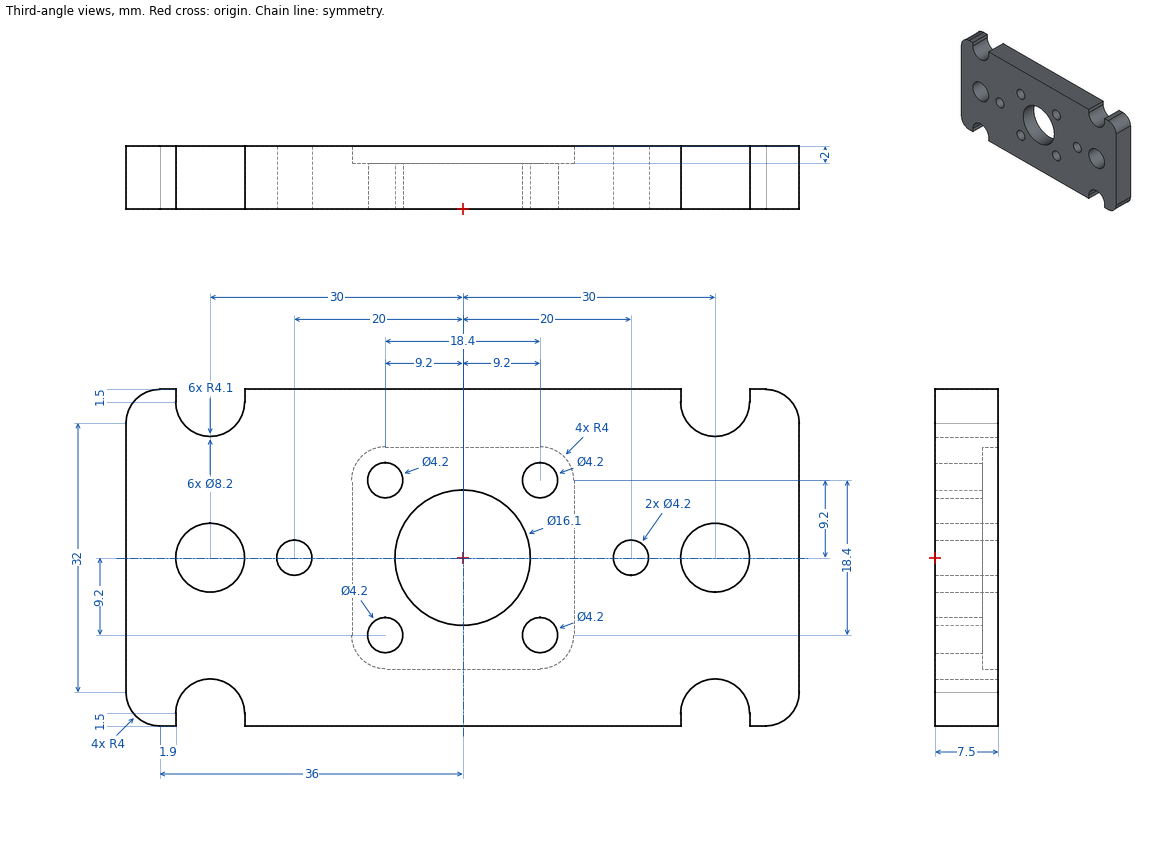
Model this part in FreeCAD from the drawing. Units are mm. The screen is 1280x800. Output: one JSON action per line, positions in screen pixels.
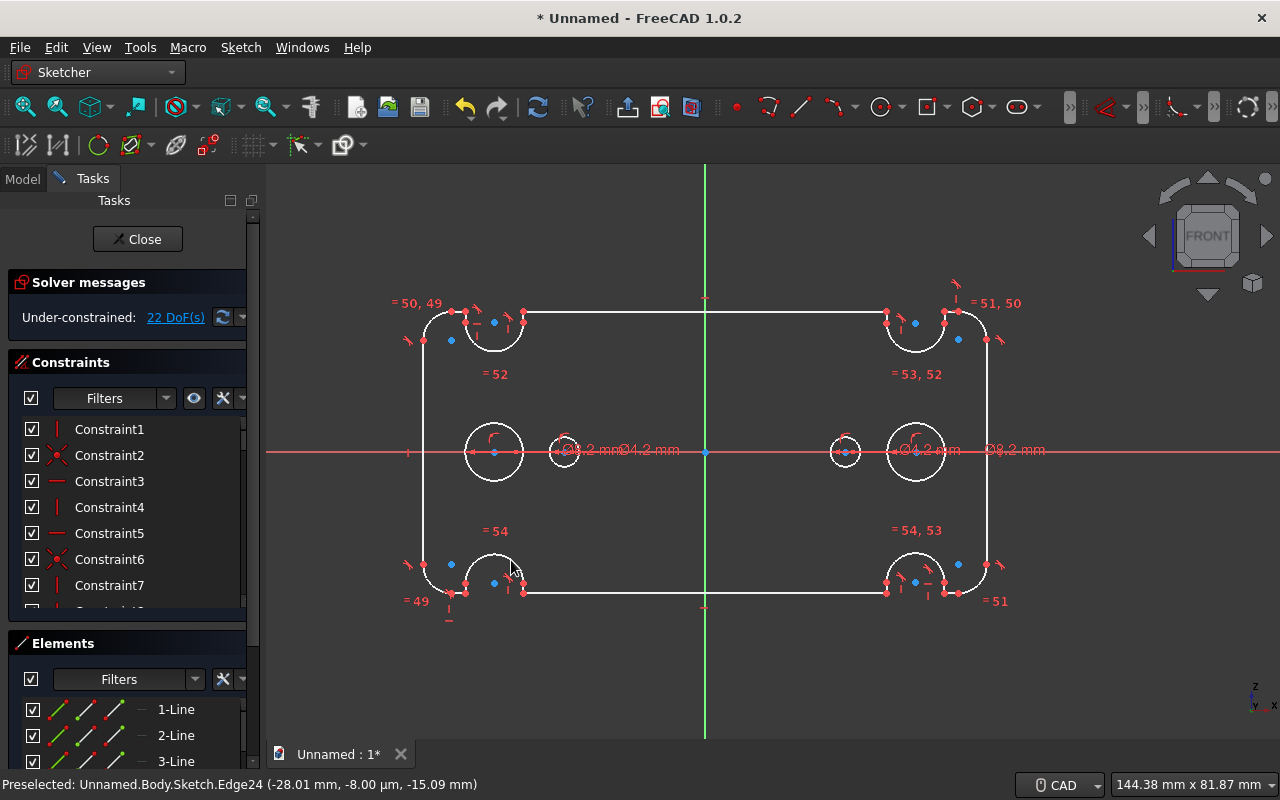
{"action": "left_click", "coordinate": [494, 323]}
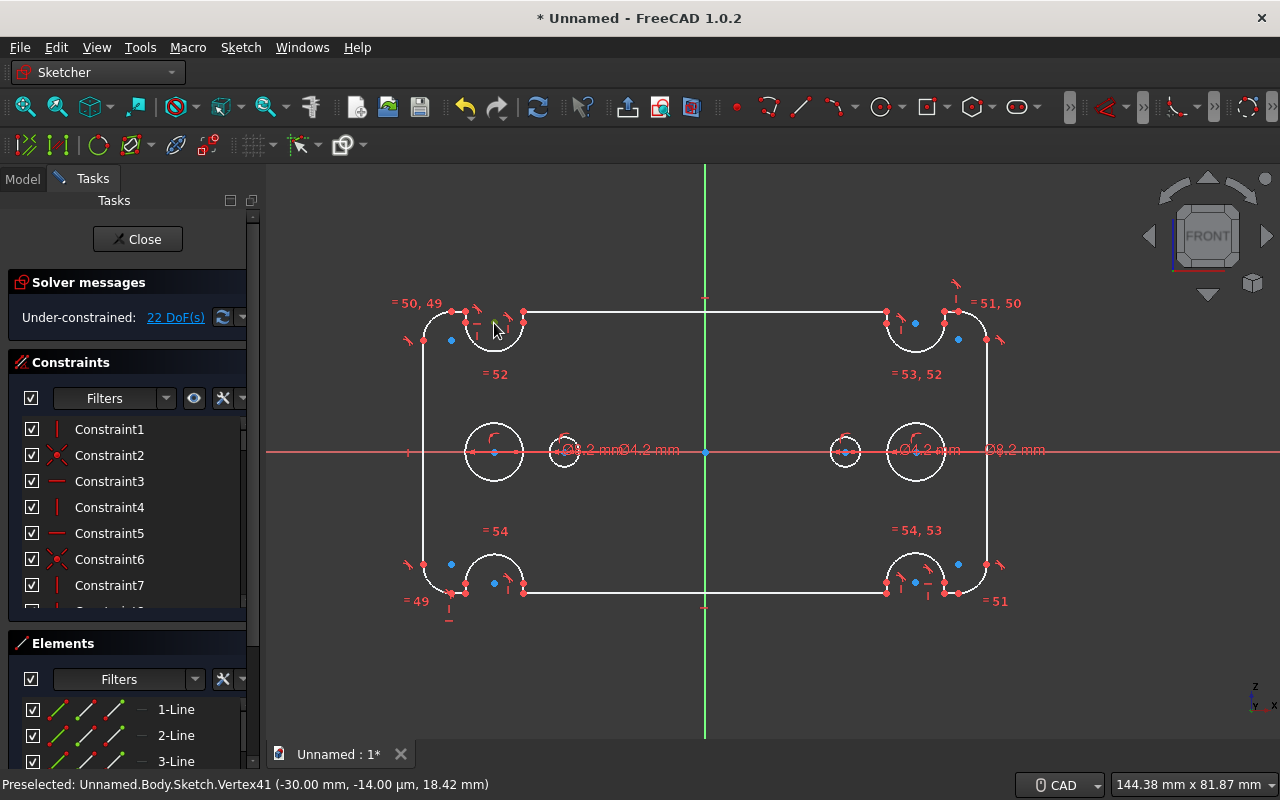
{"action": "left_click", "coordinate": [916, 323]}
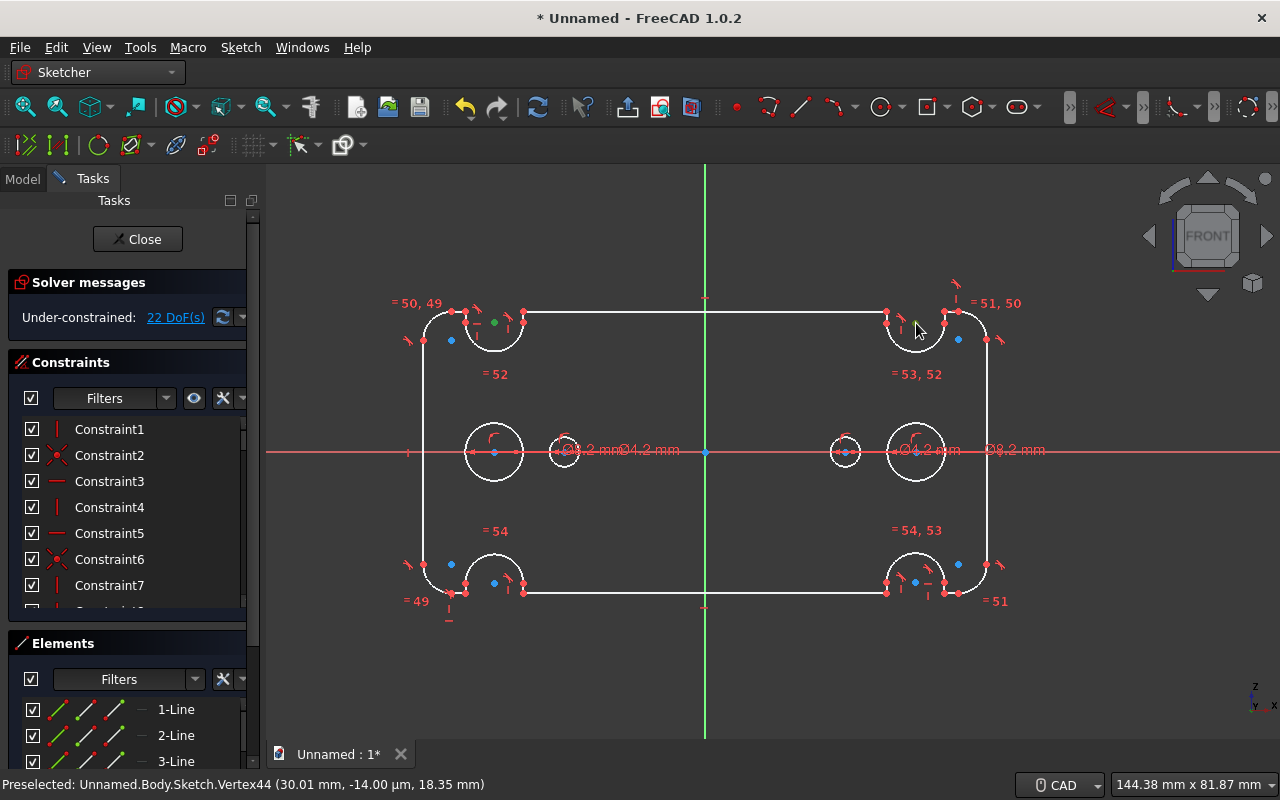
{"action": "left_click", "coordinate": [705, 674]}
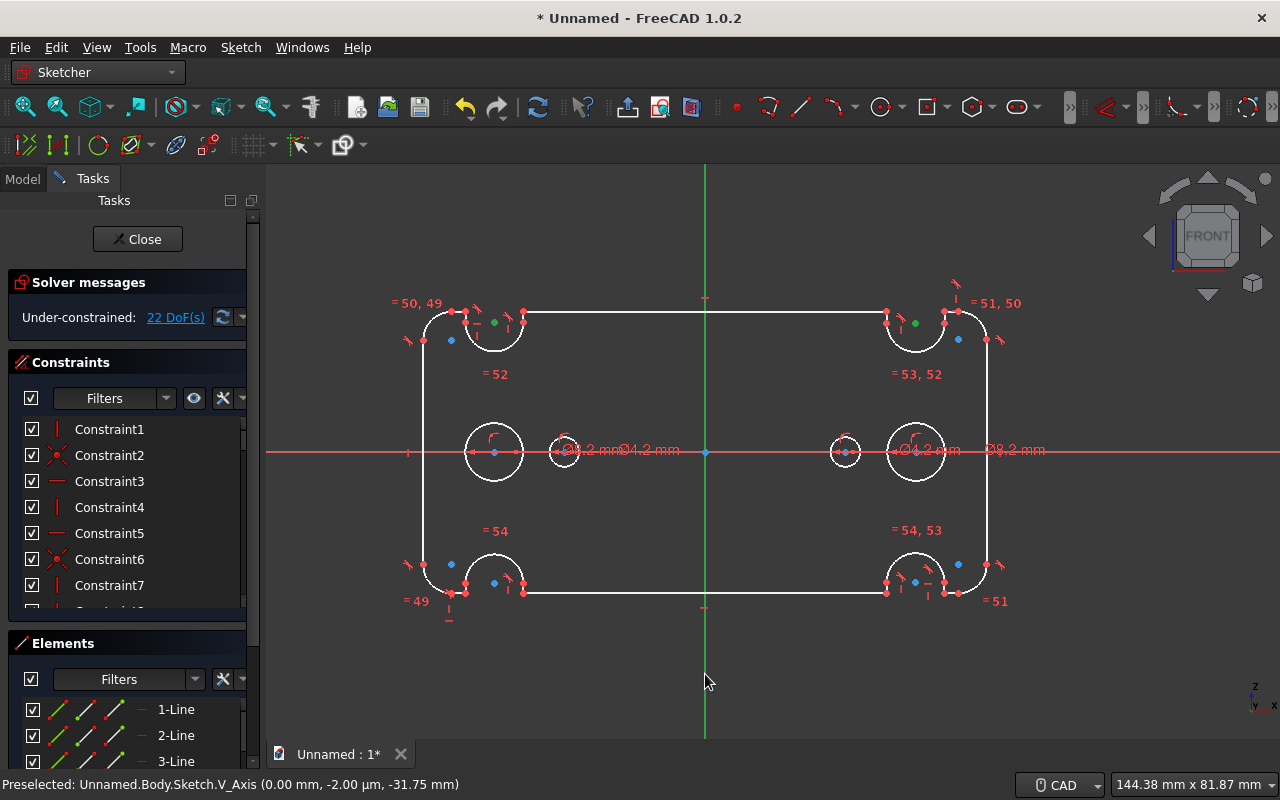
{"action": "key", "text": "s"}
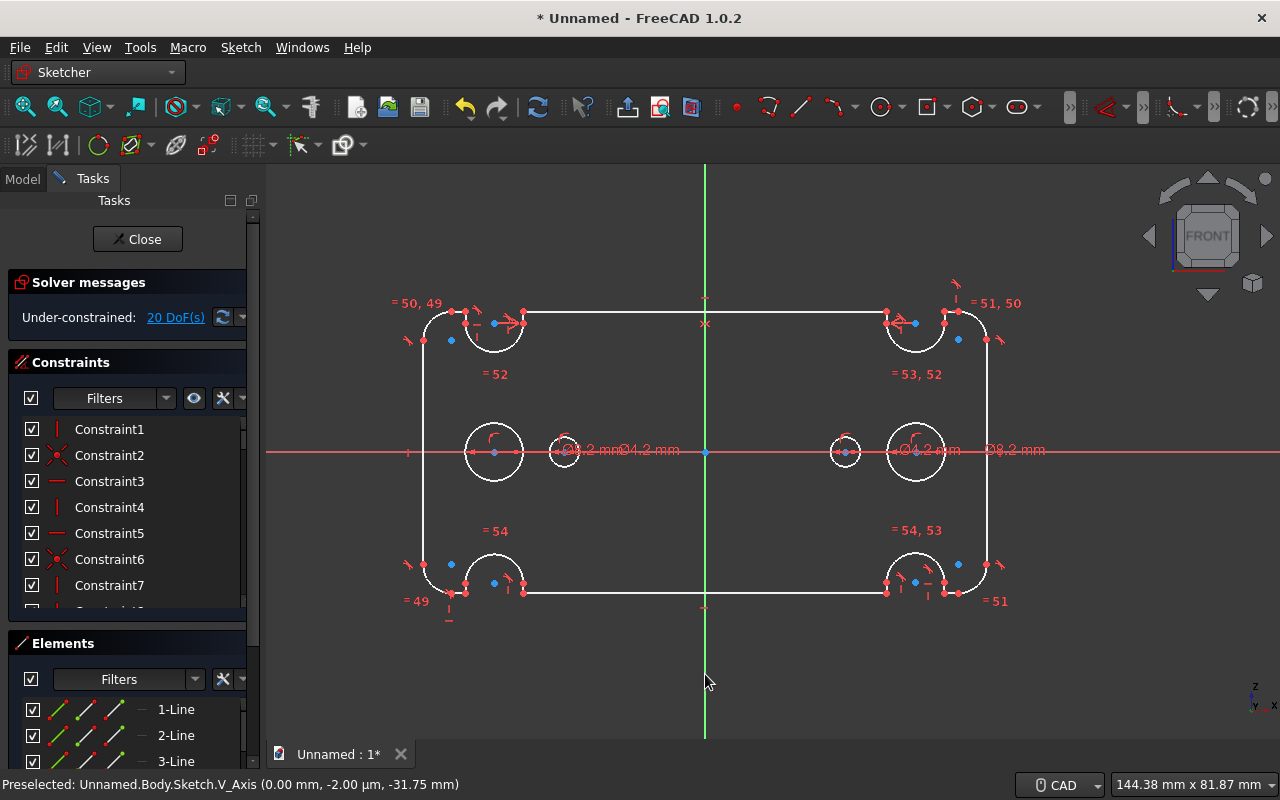
{"action": "left_click", "coordinate": [452, 340]}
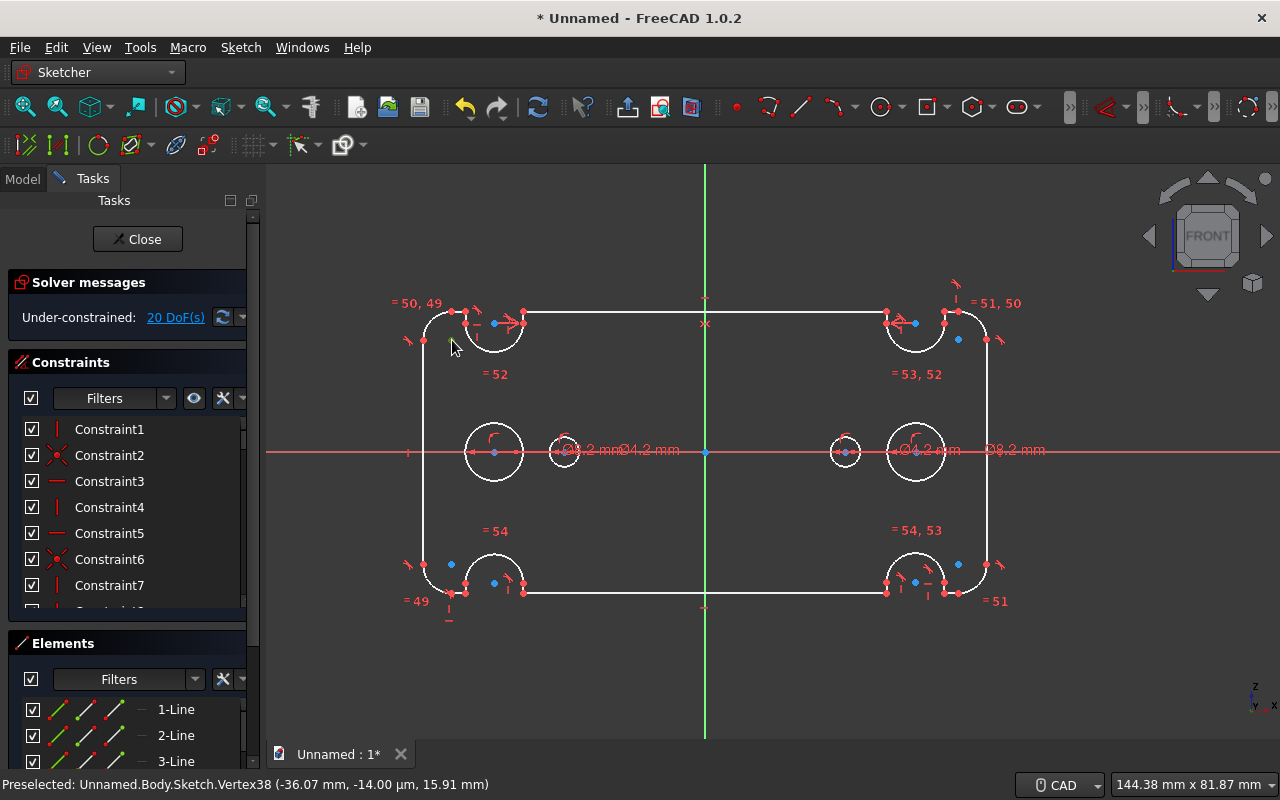
{"action": "left_click", "coordinate": [958, 340]}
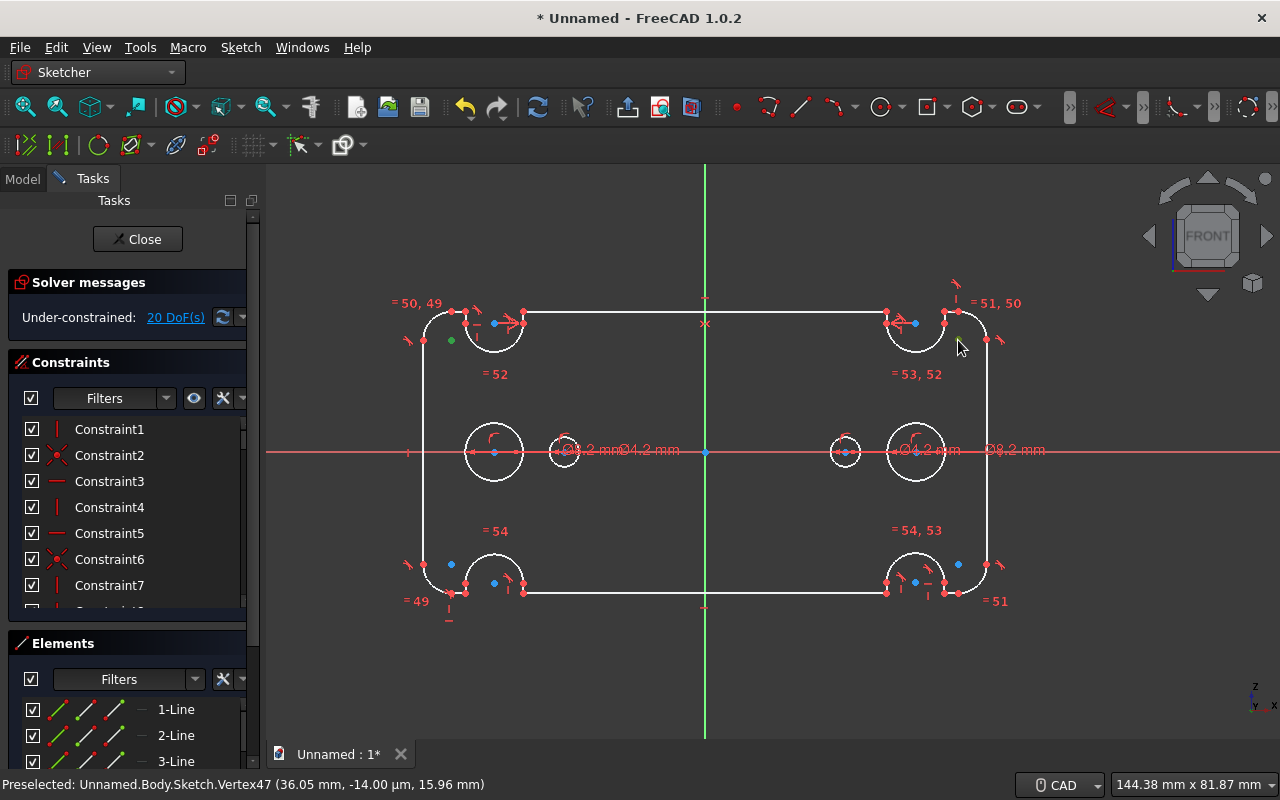
{"action": "left_click", "coordinate": [705, 674]}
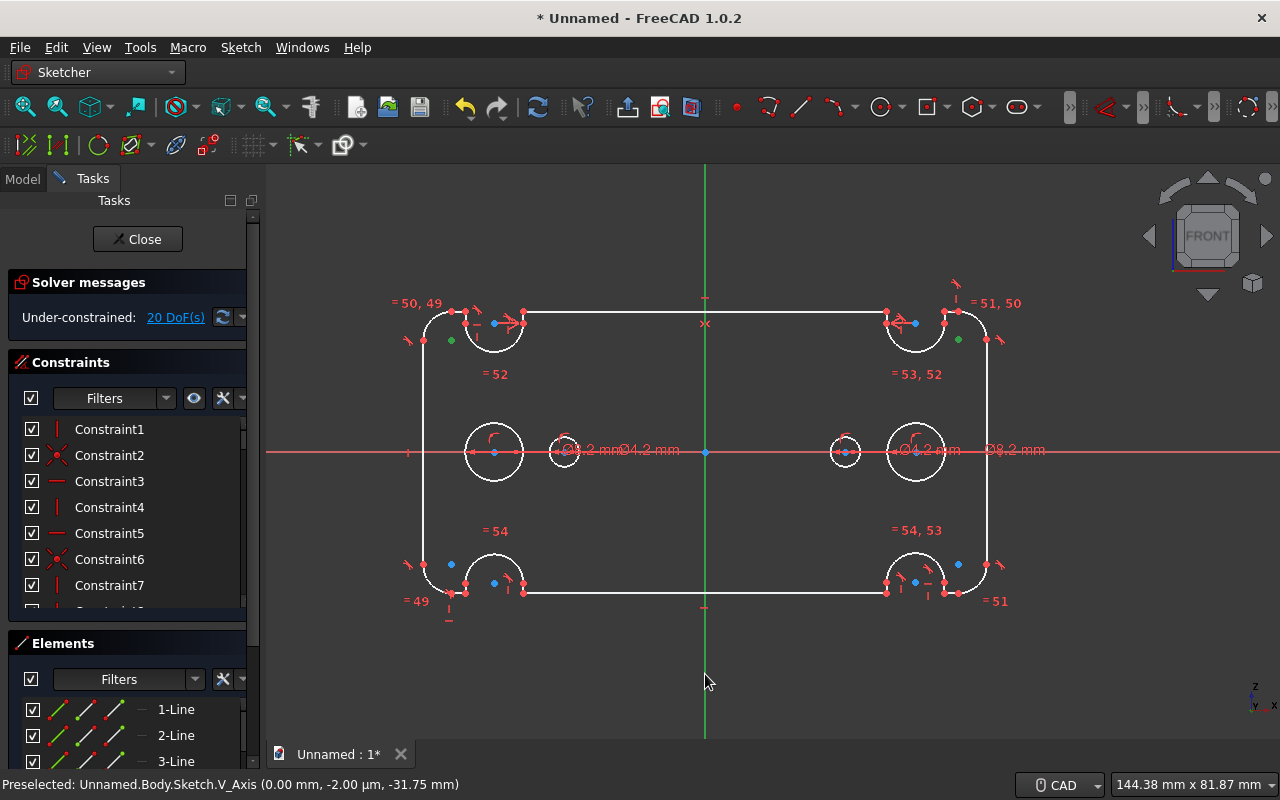
{"action": "key", "text": "s"}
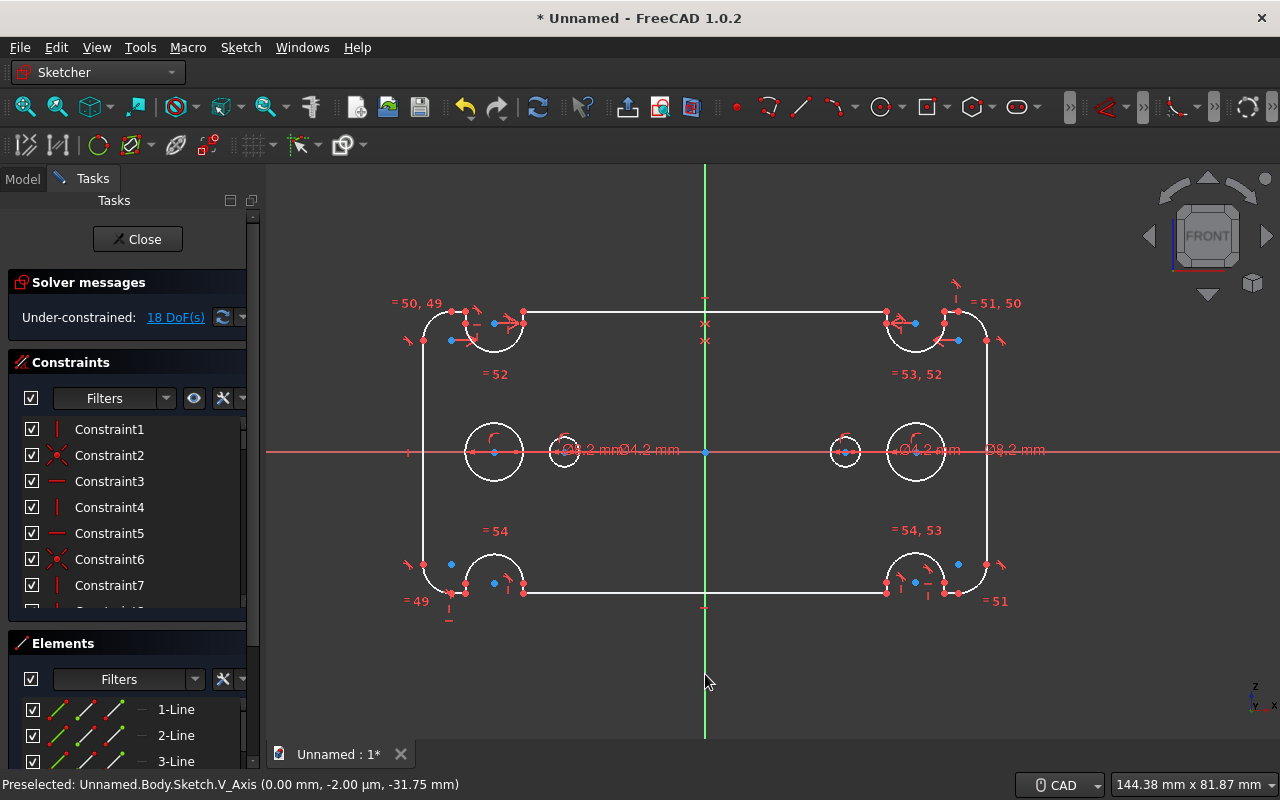
{"action": "left_click", "coordinate": [916, 323]}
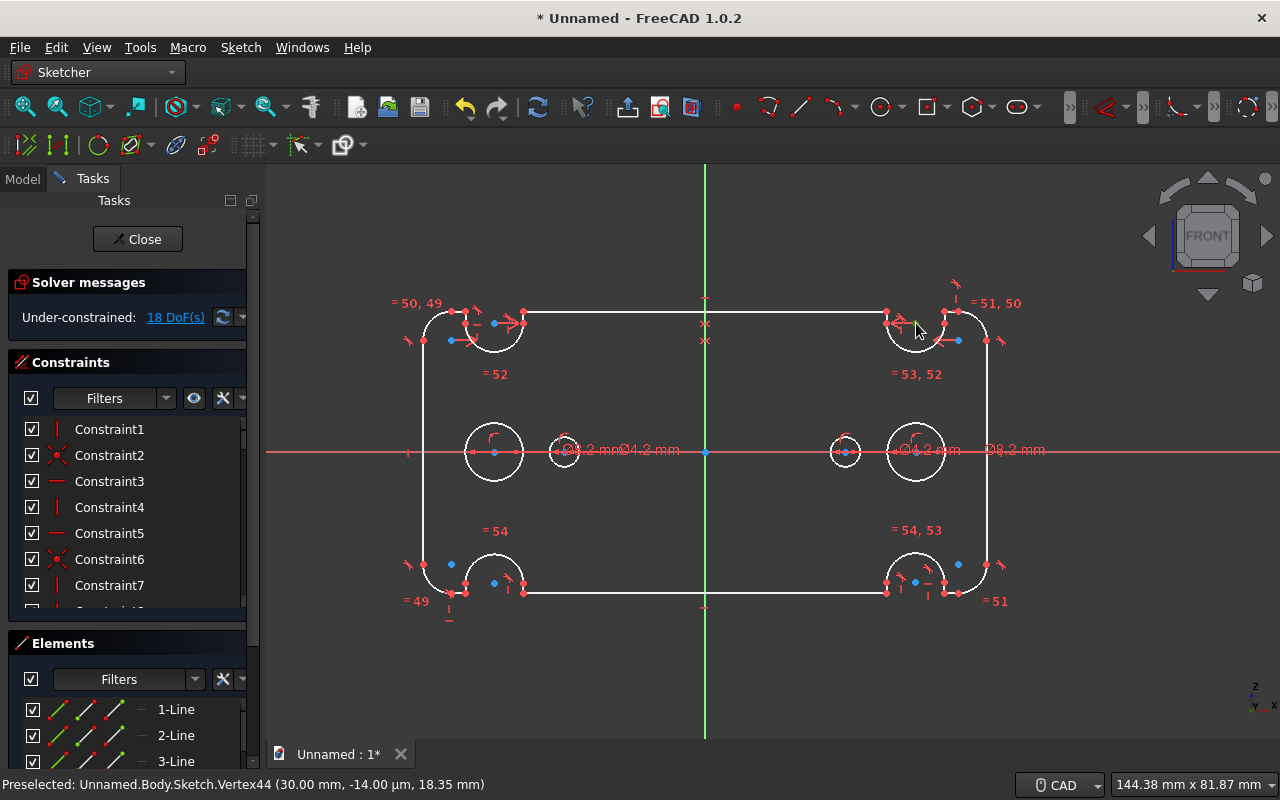
{"action": "left_click", "coordinate": [916, 582]}